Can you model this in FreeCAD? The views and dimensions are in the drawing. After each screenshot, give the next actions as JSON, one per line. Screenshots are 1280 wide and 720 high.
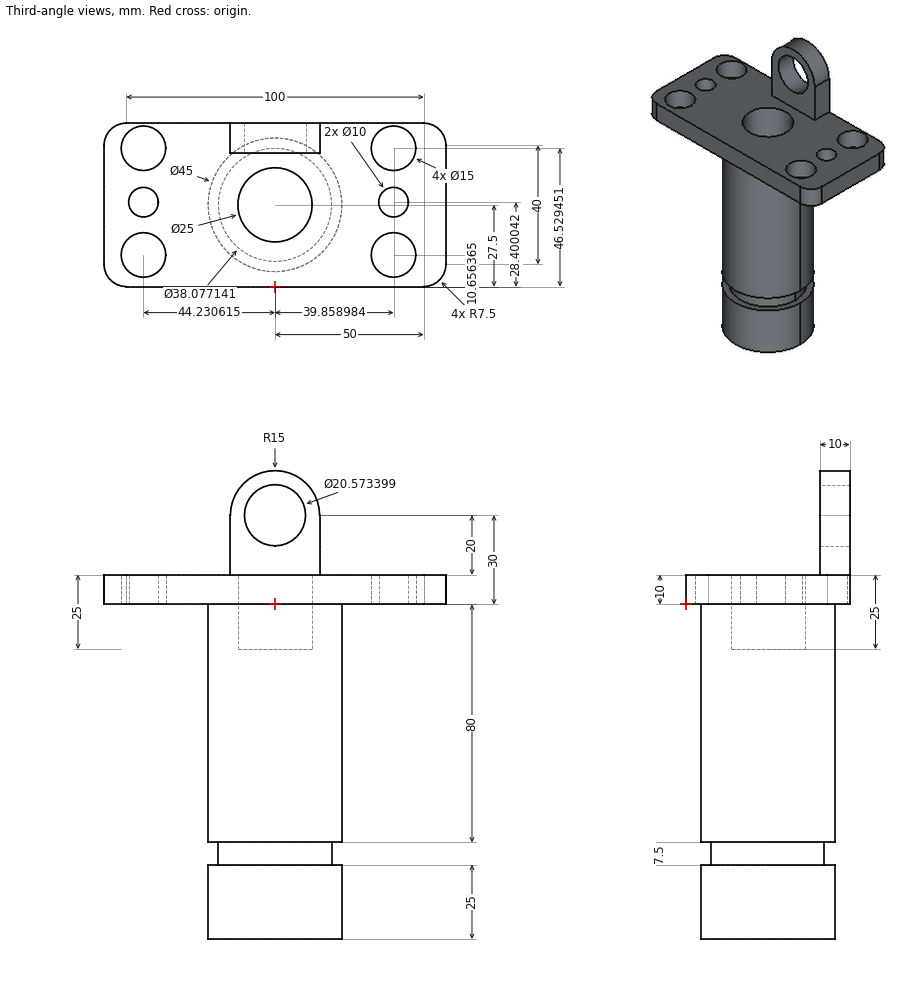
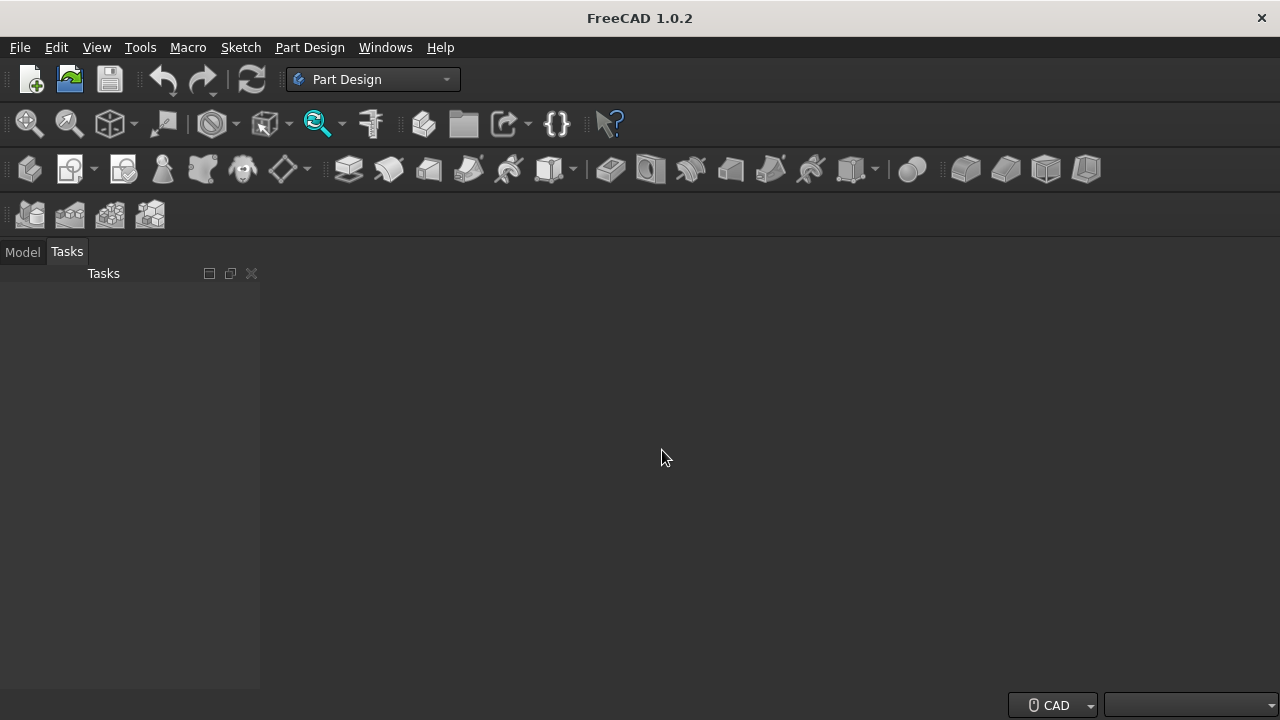
{"action": "left_click", "coordinate": [30, 80]}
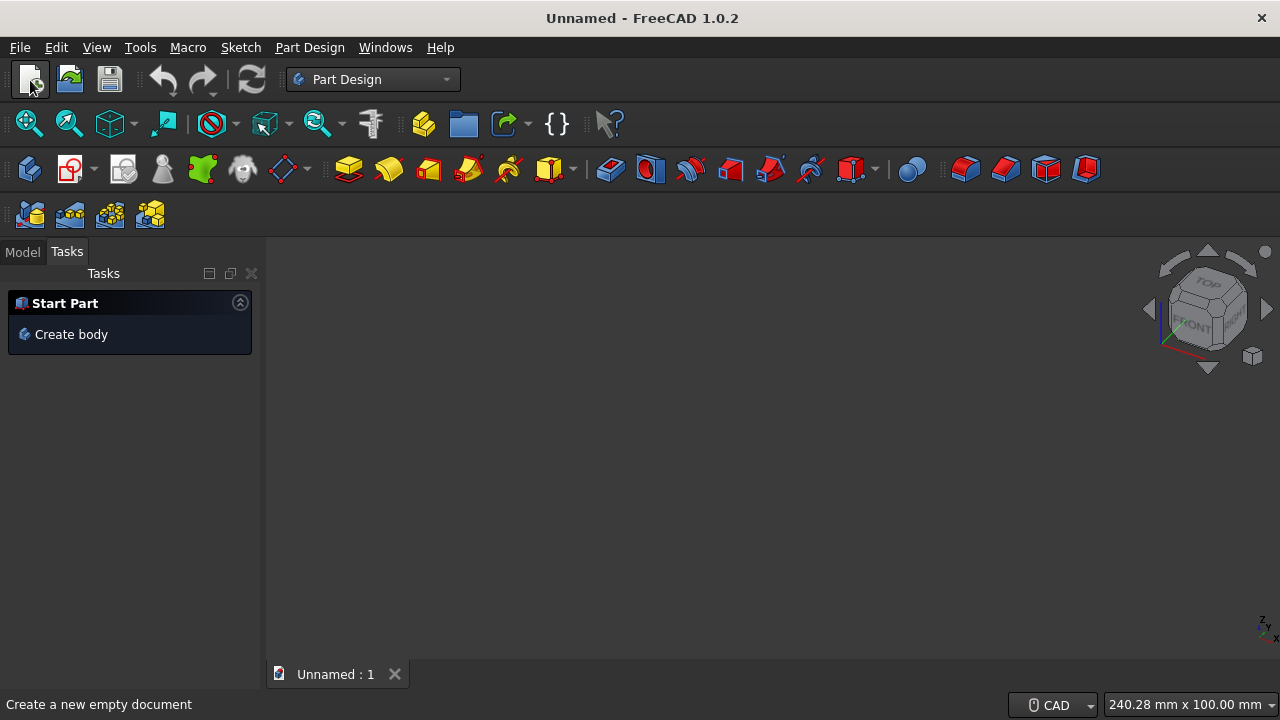
{"action": "left_click", "coordinate": [70, 170]}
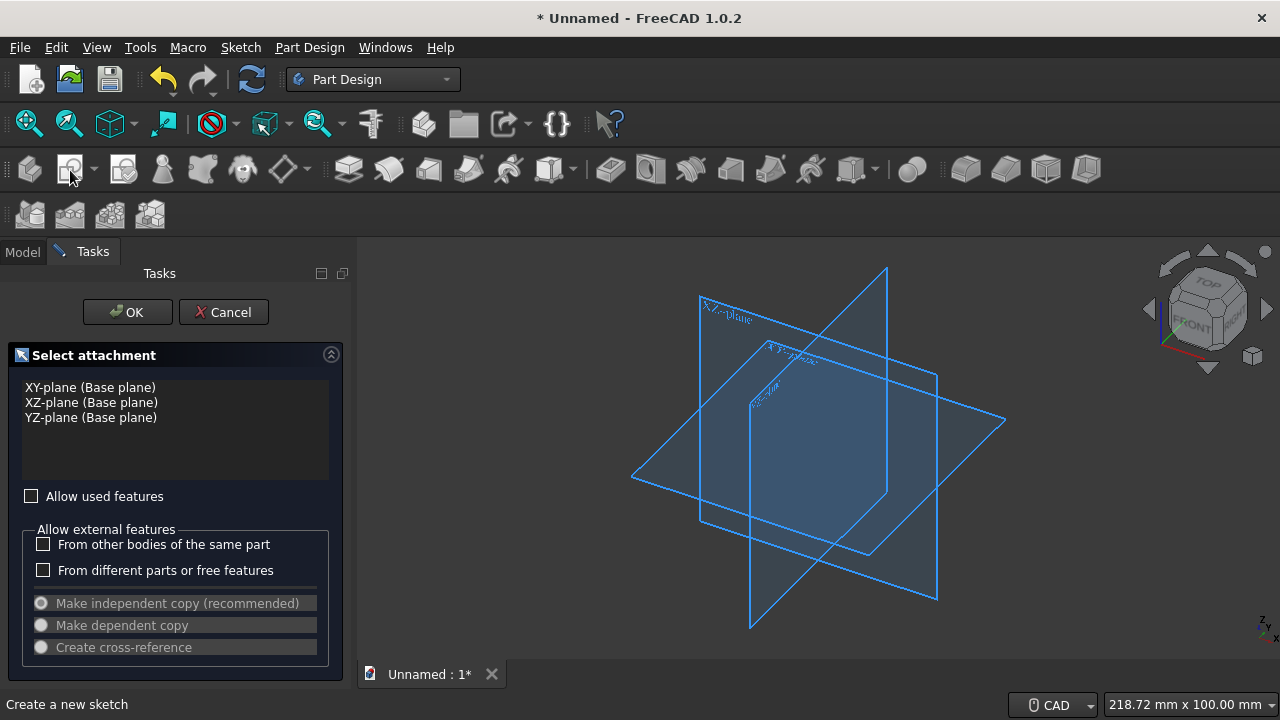
{"action": "left_click", "coordinate": [82, 388]}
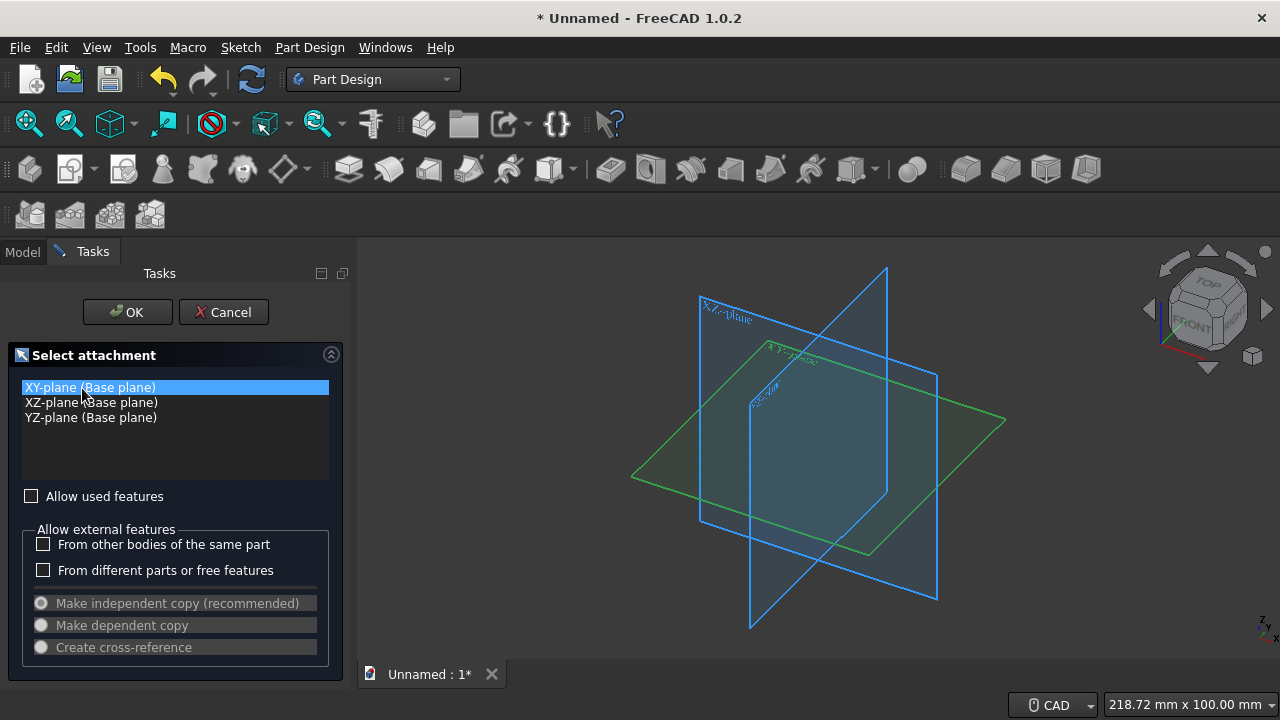
{"action": "left_click", "coordinate": [128, 312]}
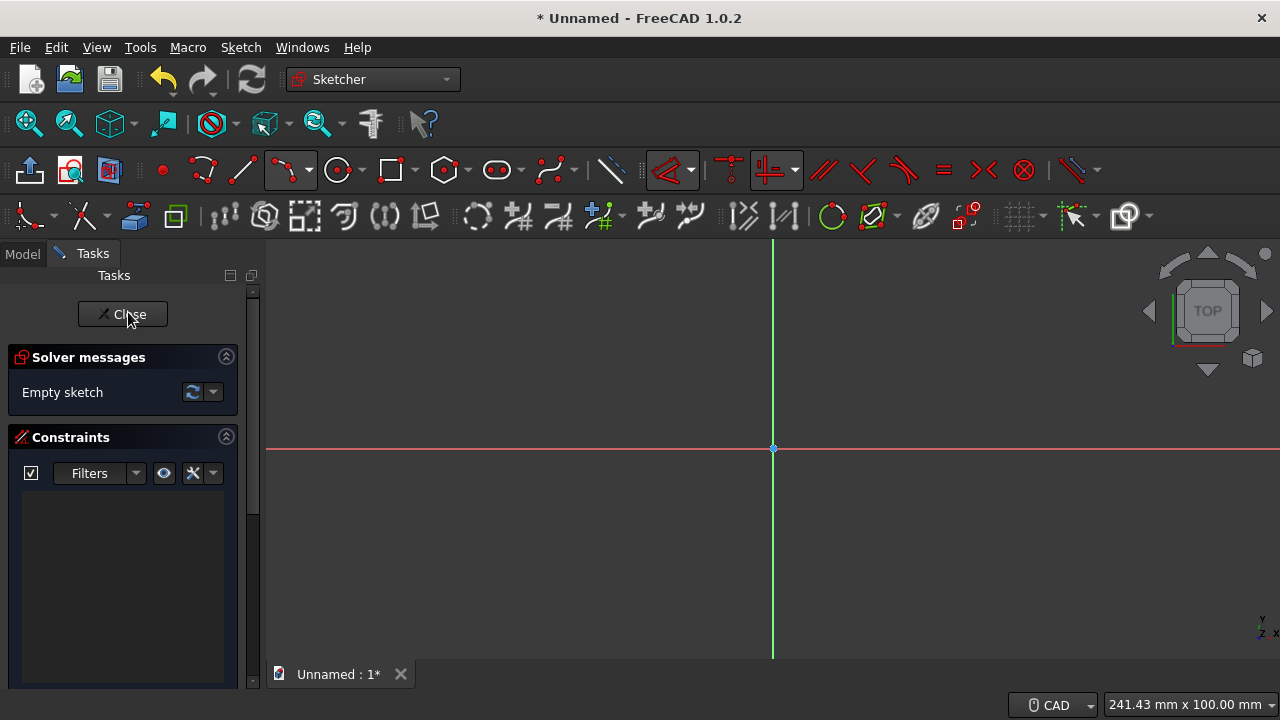
{"action": "scroll", "coordinate": [395, 631], "scroll_direction": "down", "scroll_amount": 1}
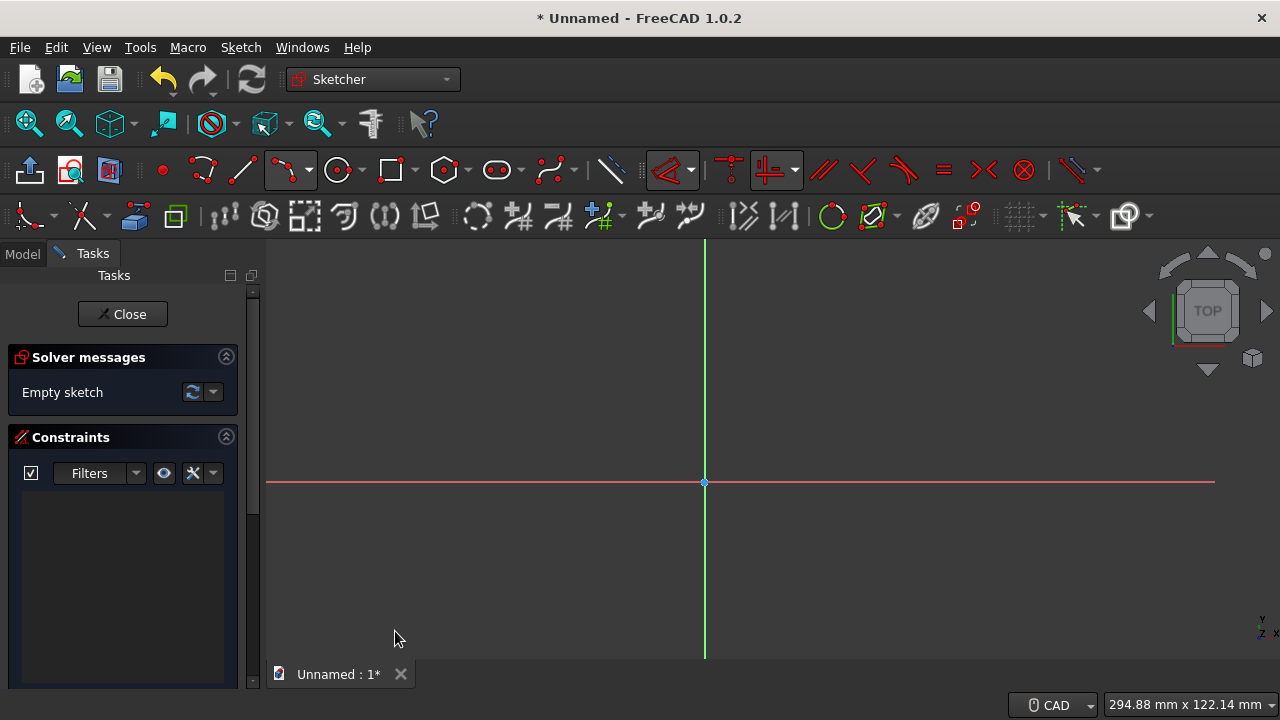
{"action": "scroll", "coordinate": [705, 267], "scroll_direction": "up", "scroll_amount": 2}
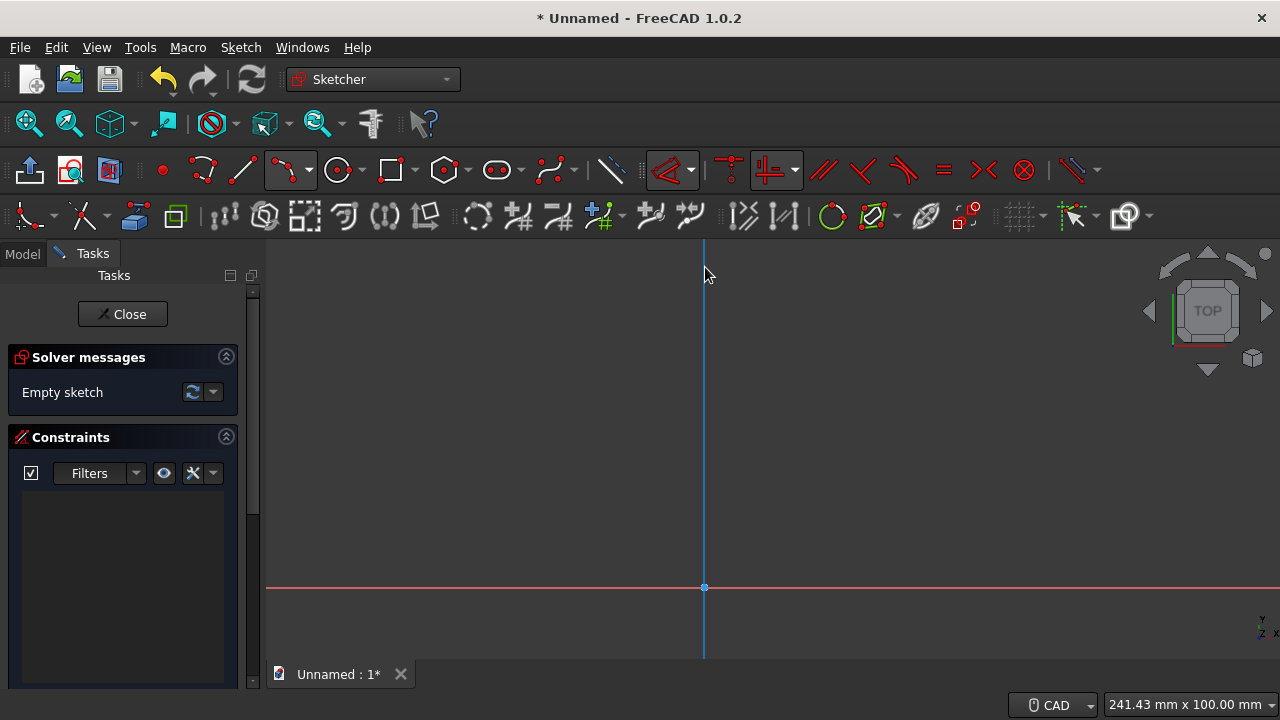
{"action": "left_click", "coordinate": [244, 170]}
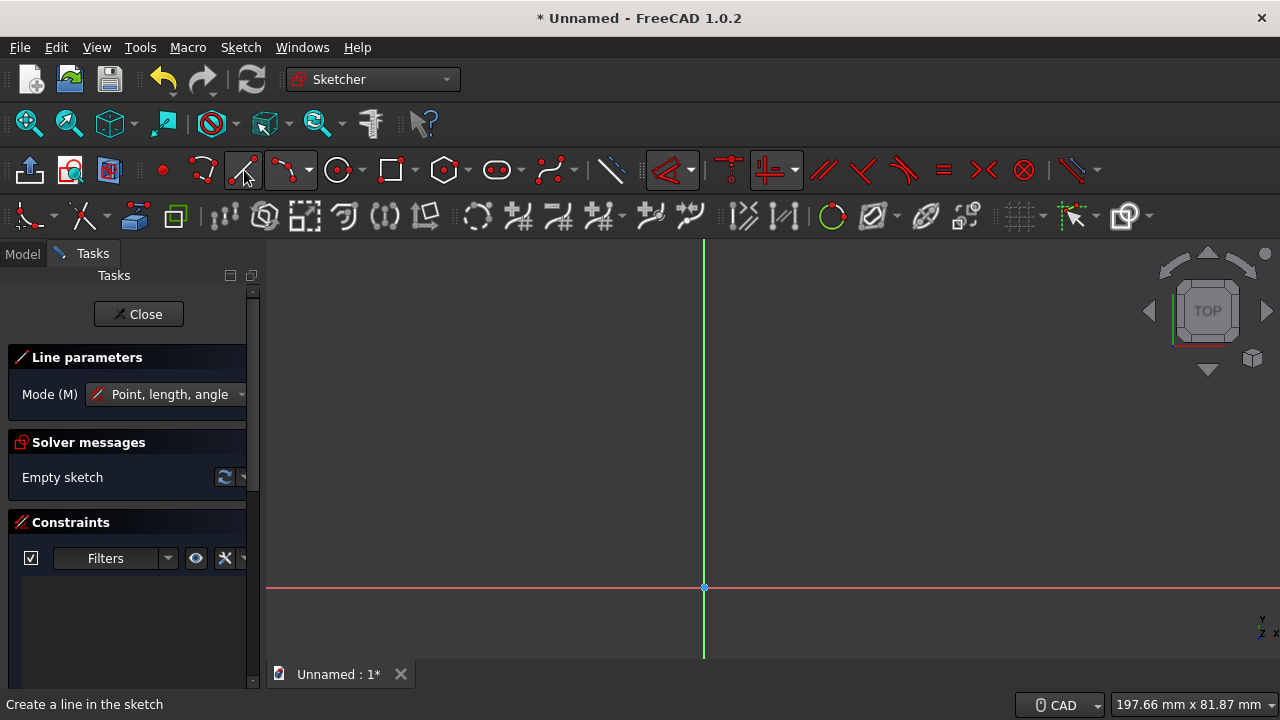
{"action": "left_click", "coordinate": [999, 549]}
{"action": "left_click", "coordinate": [999, 344]}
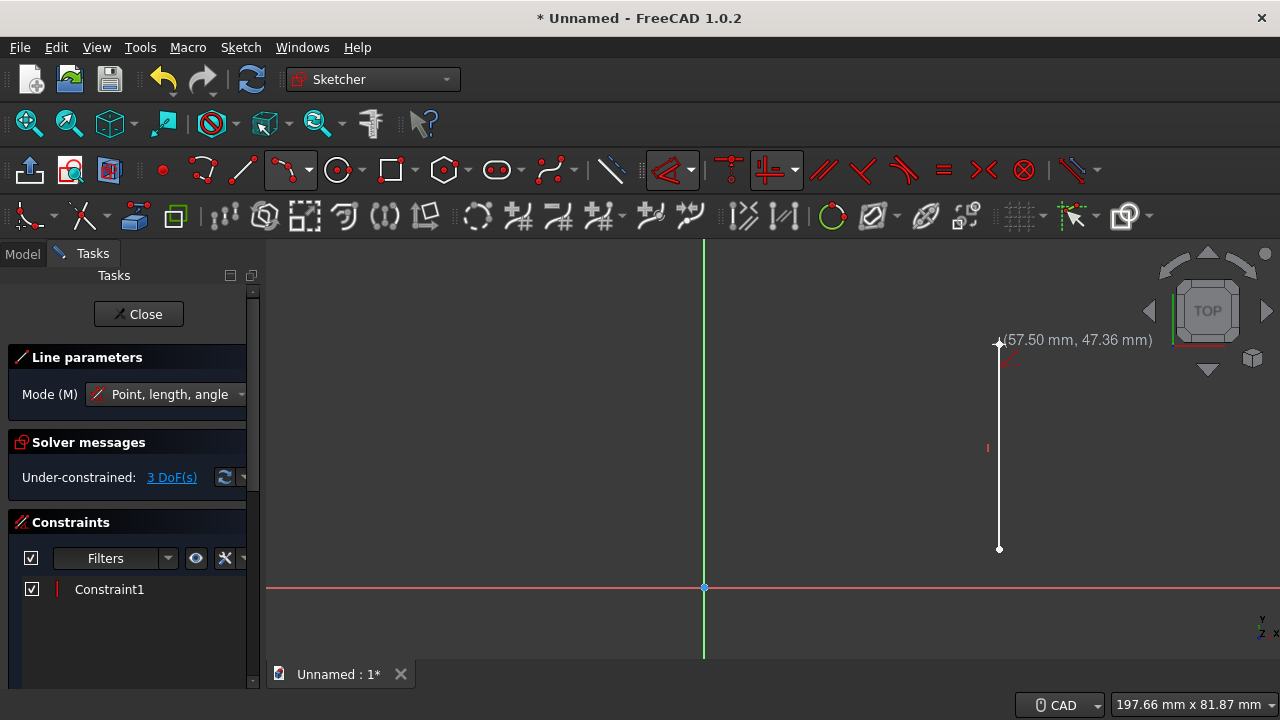
{"action": "left_click", "coordinate": [961, 306]}
{"action": "left_click", "coordinate": [448, 306]}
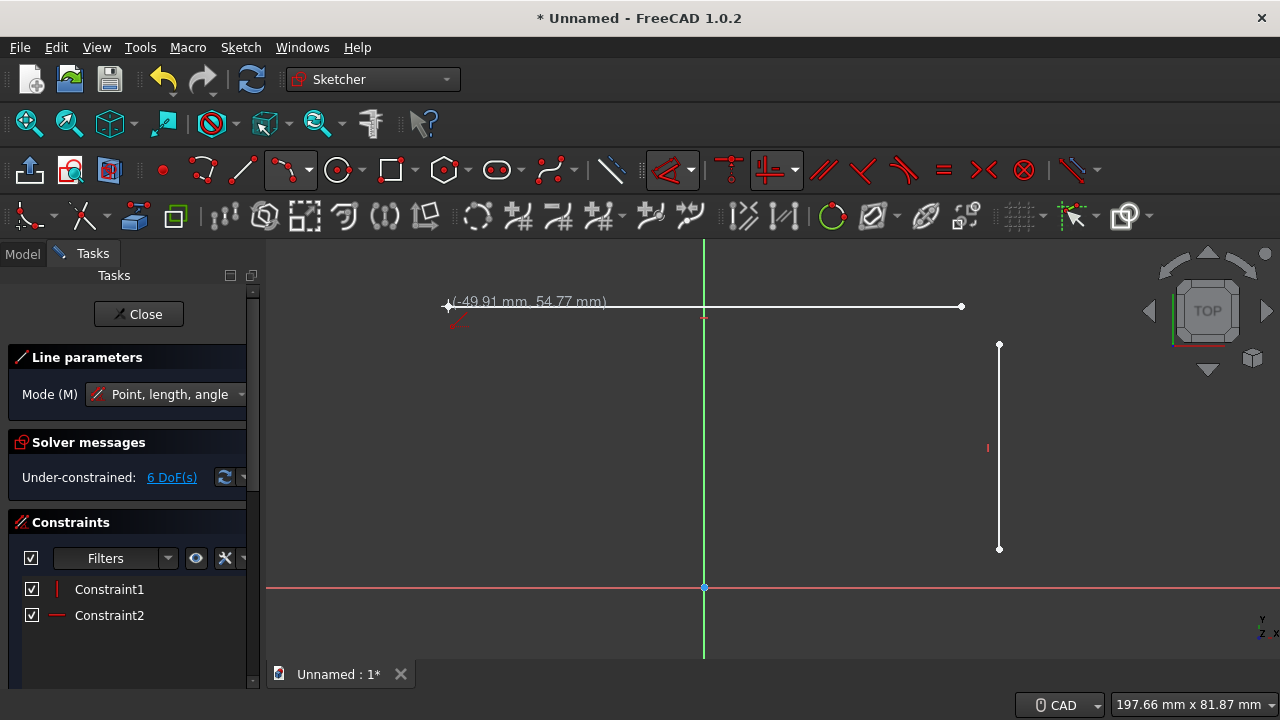
{"action": "left_click", "coordinate": [409, 344]}
{"action": "left_click", "coordinate": [409, 549]}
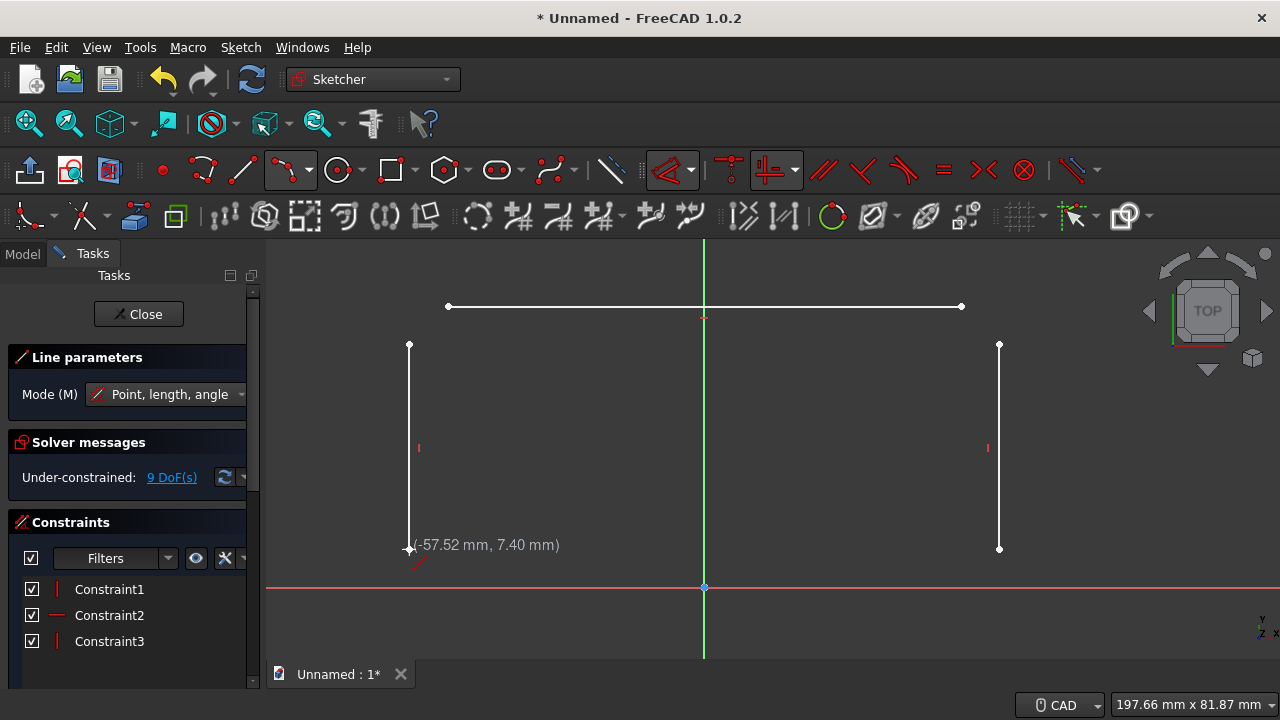
{"action": "left_click", "coordinate": [448, 588]}
{"action": "left_click", "coordinate": [961, 579]}